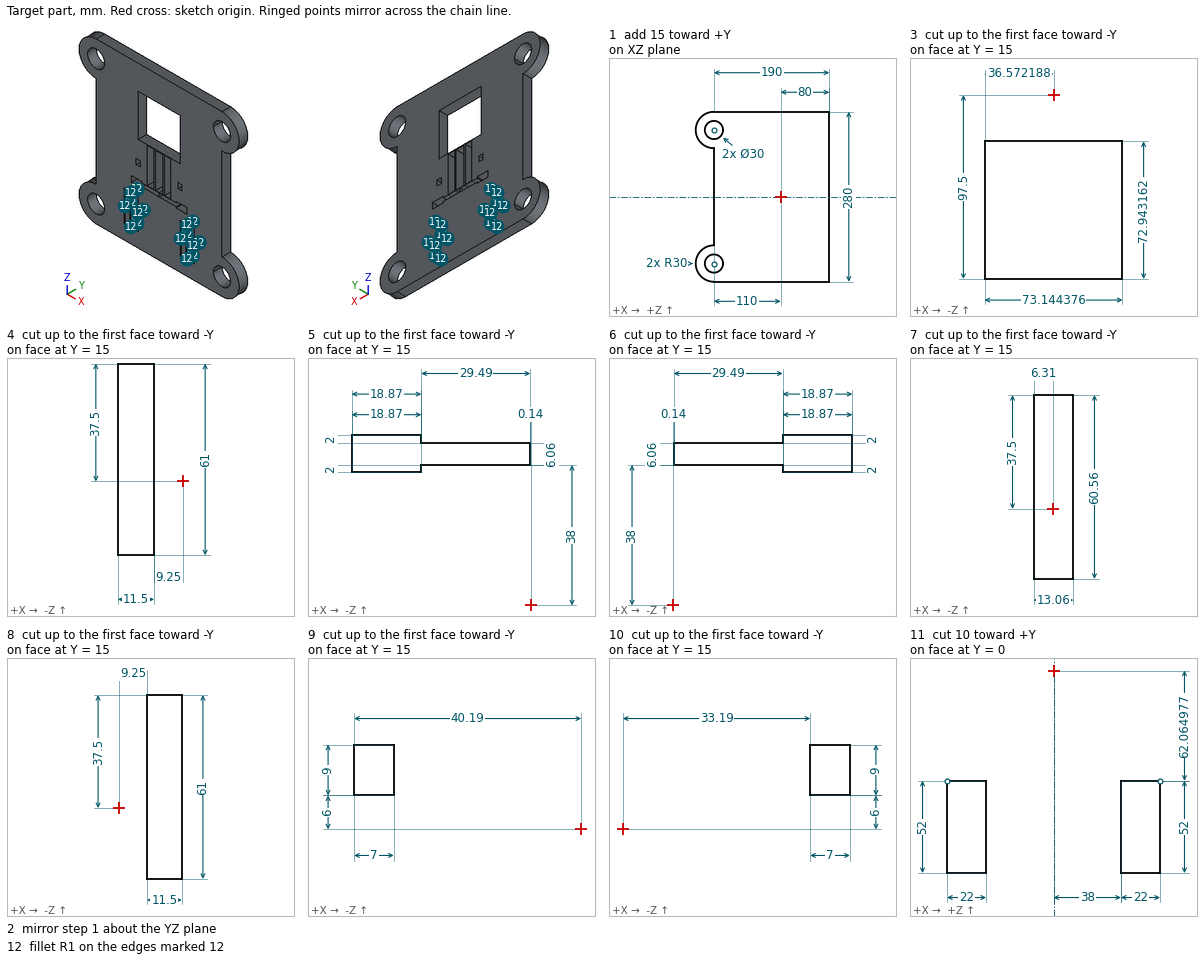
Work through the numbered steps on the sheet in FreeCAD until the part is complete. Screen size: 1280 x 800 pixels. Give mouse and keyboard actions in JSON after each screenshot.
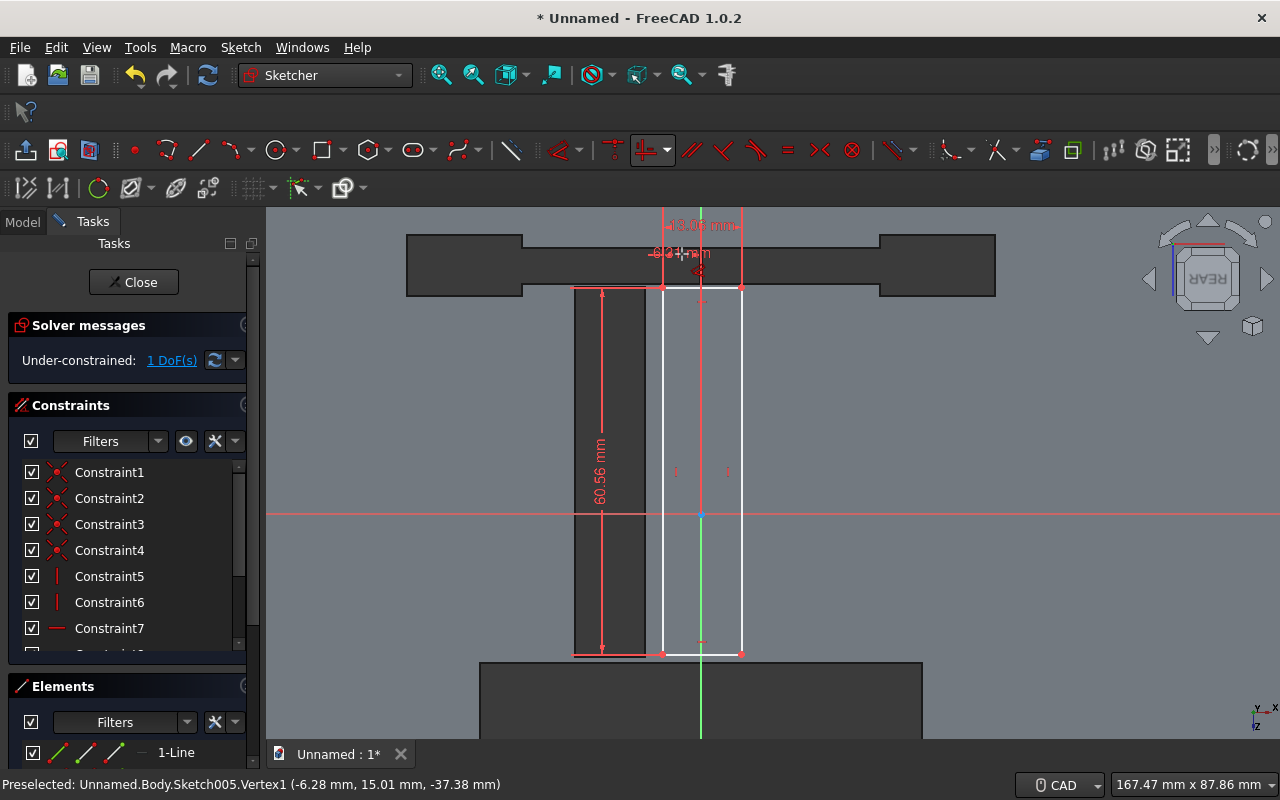
{"action": "left_click", "coordinate": [663, 288]}
{"action": "left_click", "coordinate": [629, 401]}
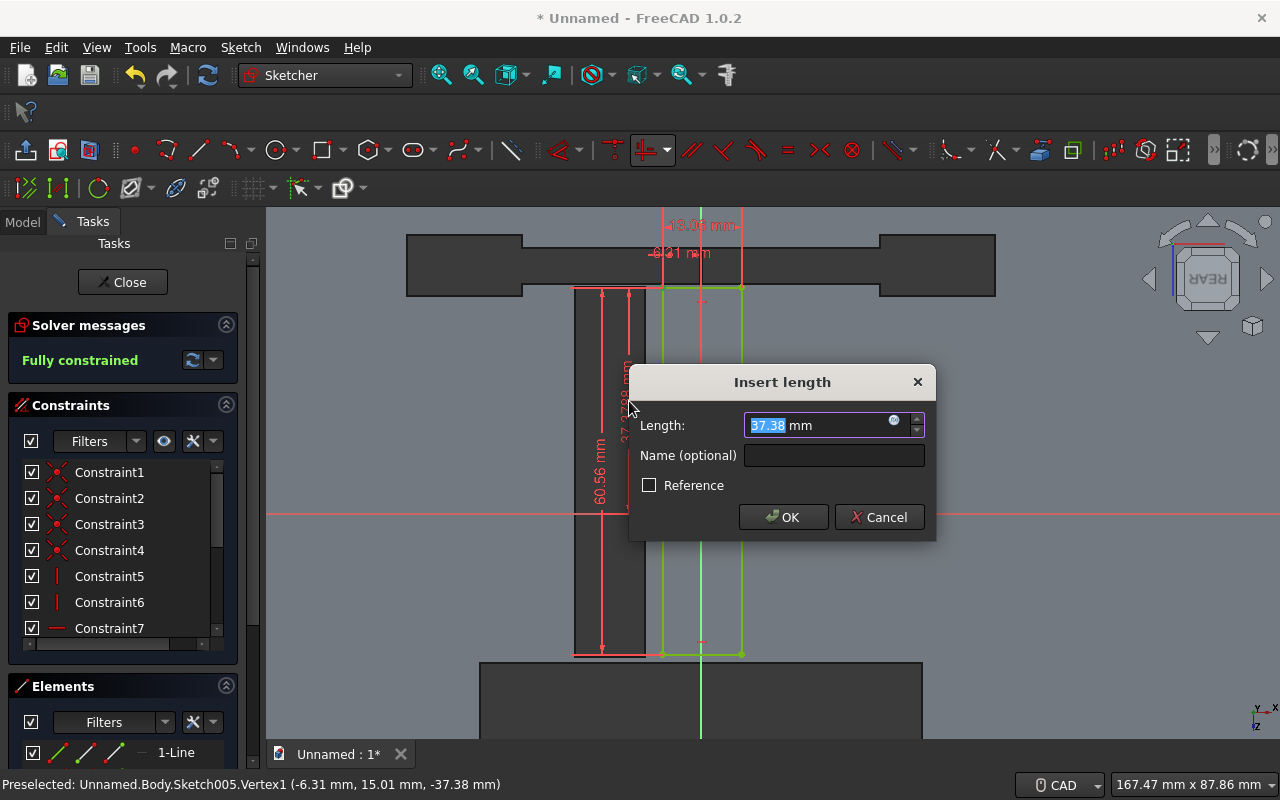
{"action": "type", "text": "37.5"}
{"action": "key", "text": "Return"}
{"action": "key", "text": "Escape"}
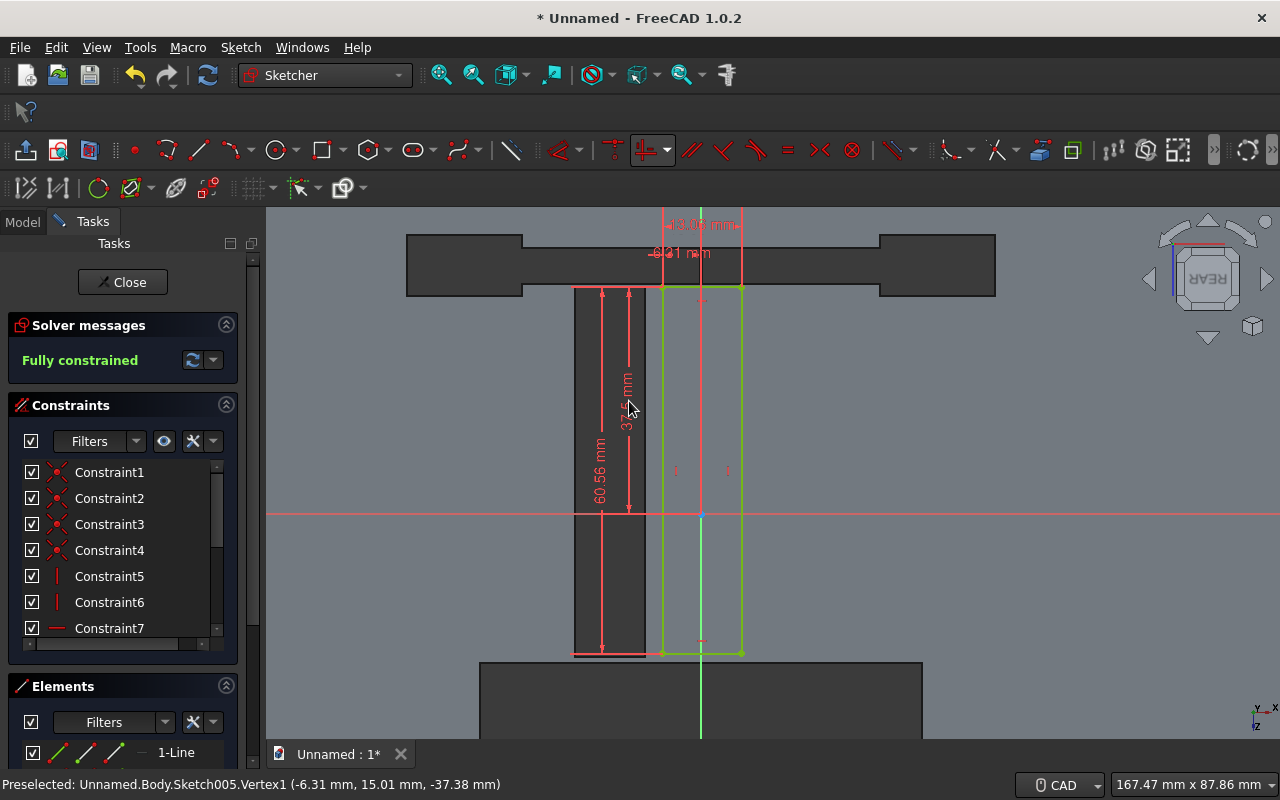
{"action": "left_click", "coordinate": [123, 282]}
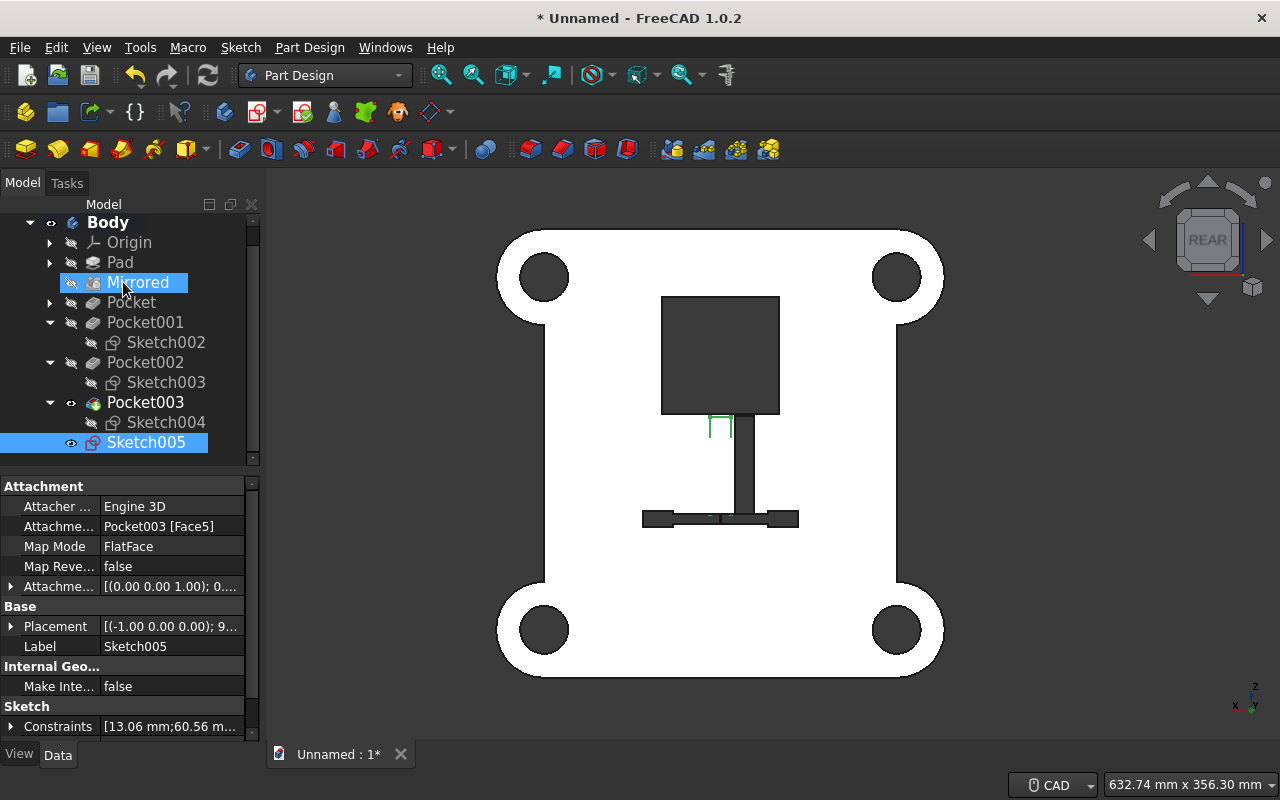
{"action": "left_click", "coordinate": [240, 150]}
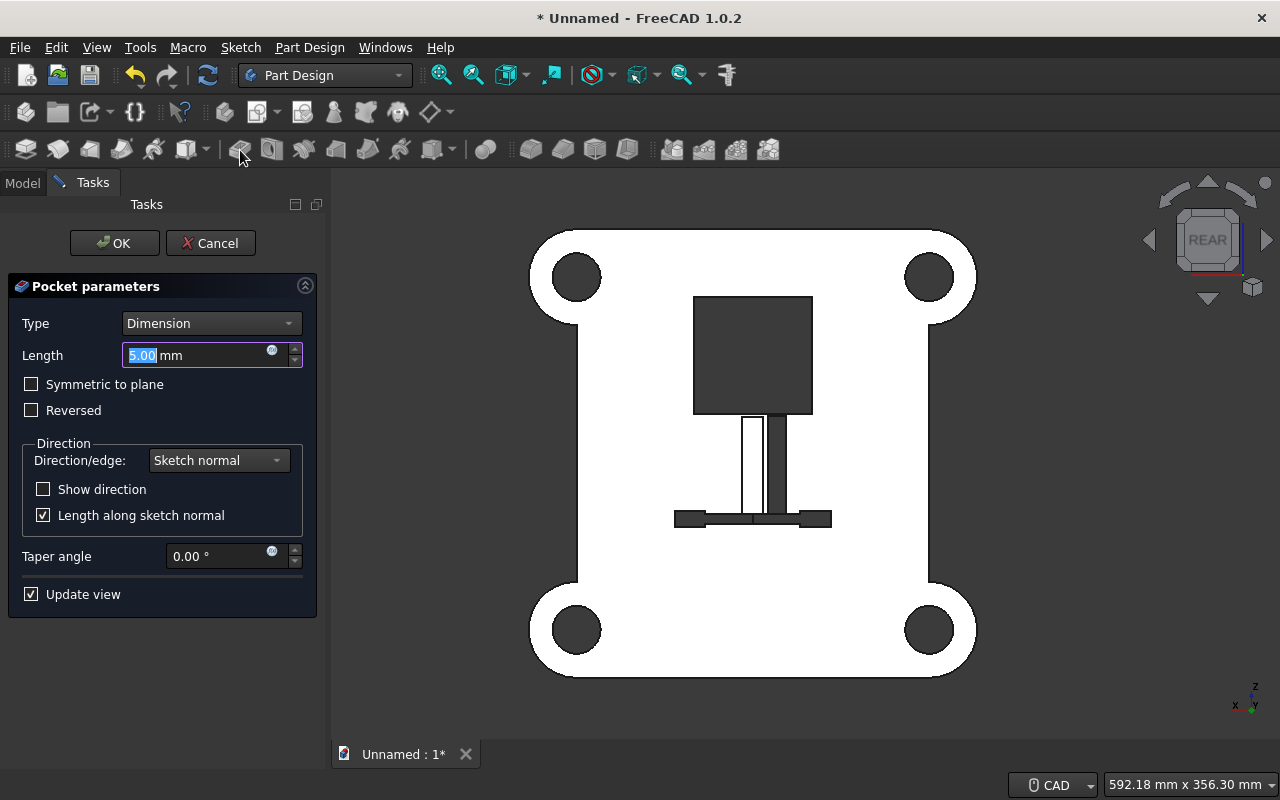
{"action": "left_click", "coordinate": [212, 324]}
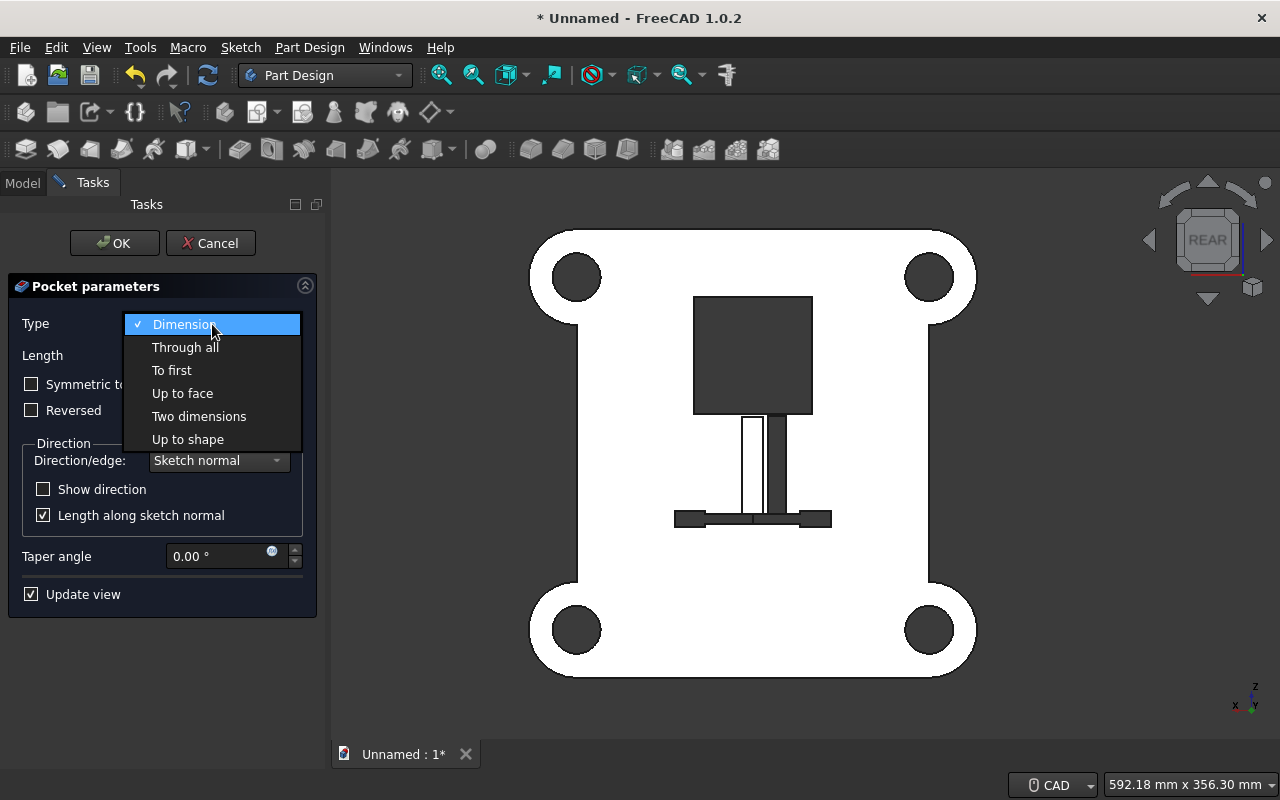
{"action": "left_click", "coordinate": [212, 370]}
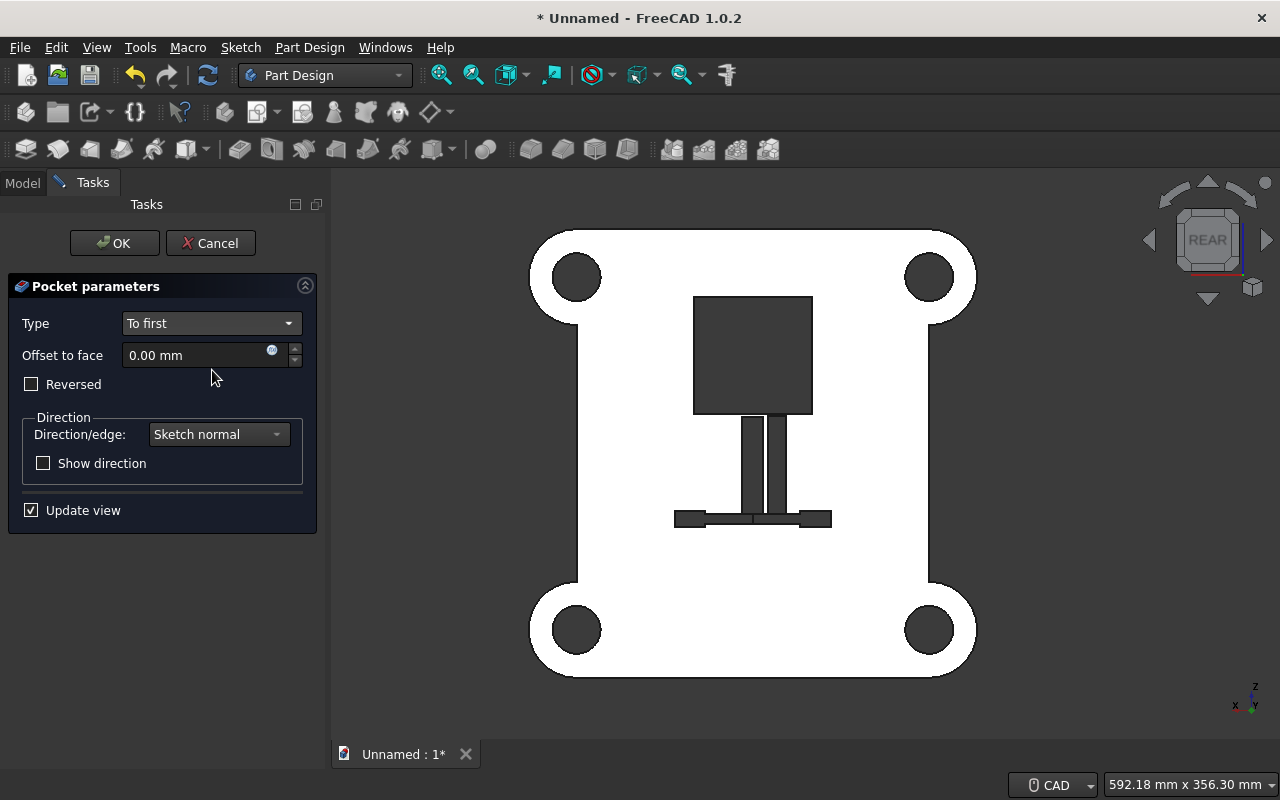
{"action": "left_click", "coordinate": [115, 243]}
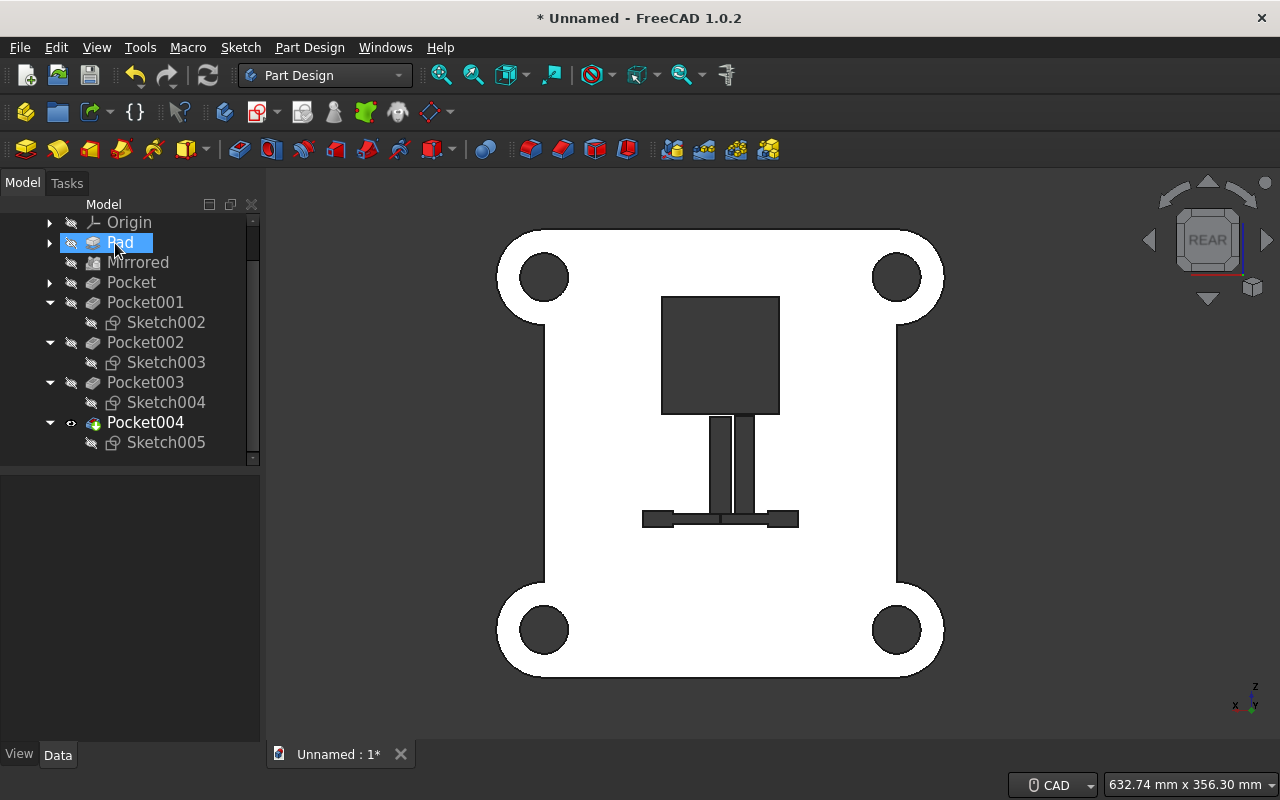
{"action": "left_click", "coordinate": [720, 581]}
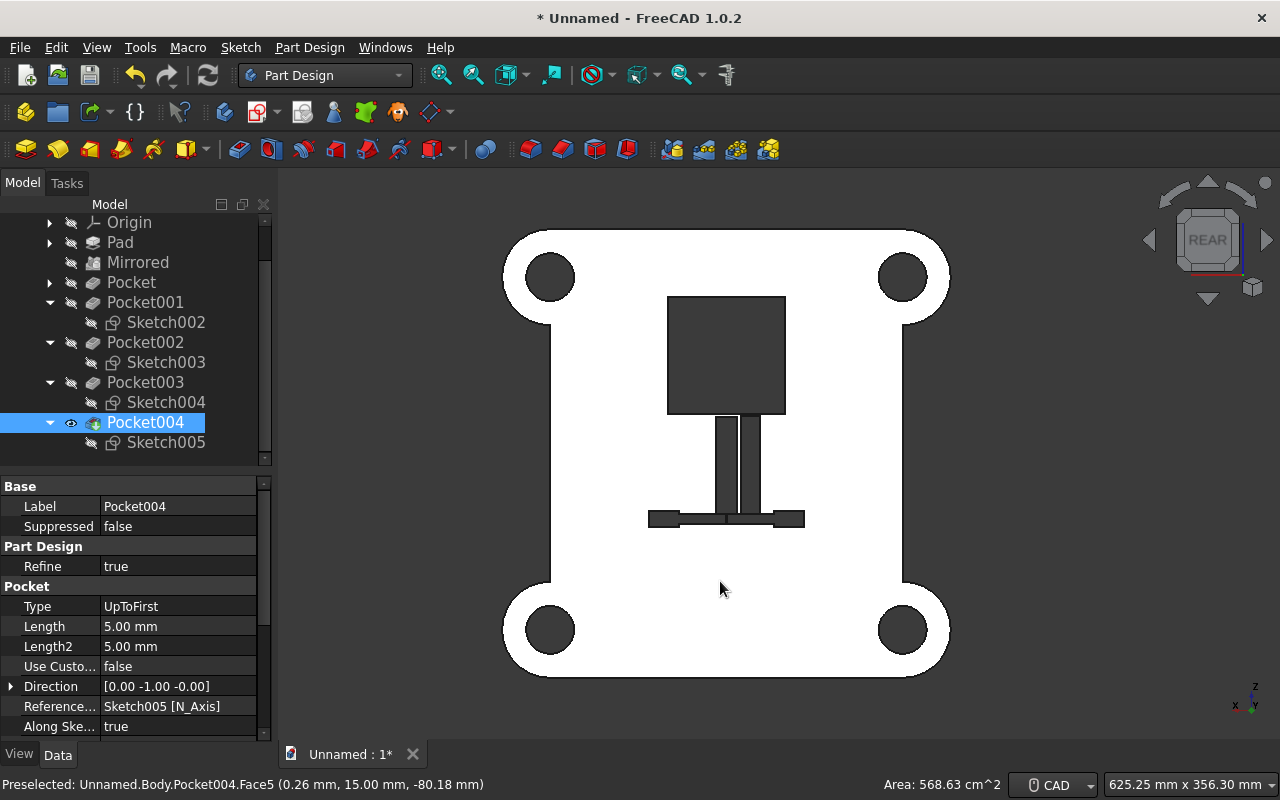
{"action": "left_click", "coordinate": [258, 112]}